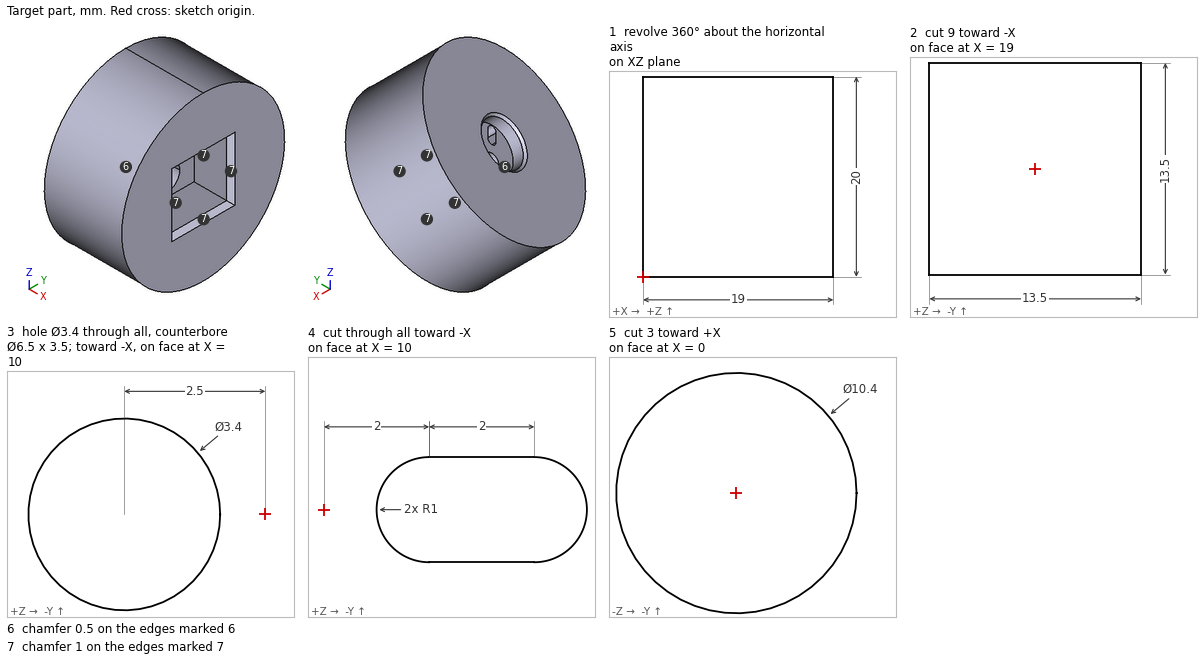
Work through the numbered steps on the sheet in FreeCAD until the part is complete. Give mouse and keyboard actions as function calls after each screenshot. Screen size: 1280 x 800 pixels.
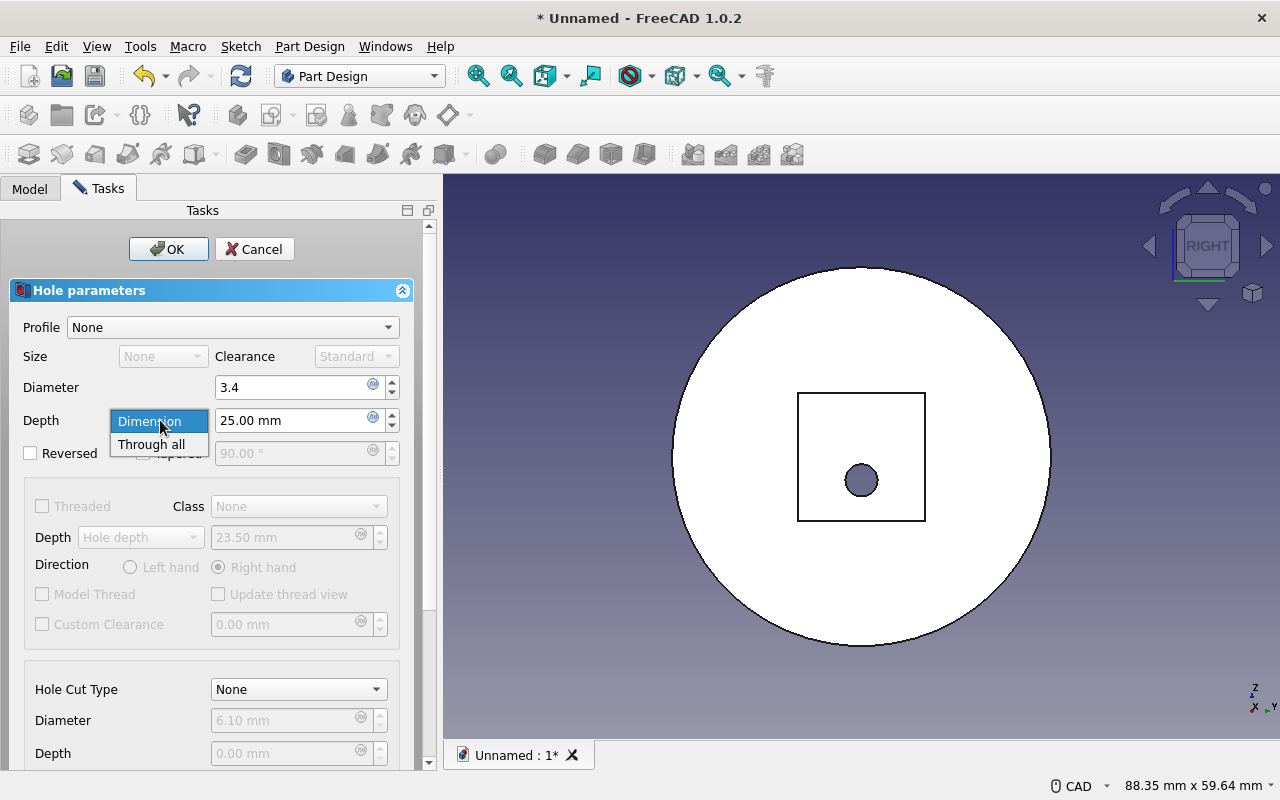
click(158, 444)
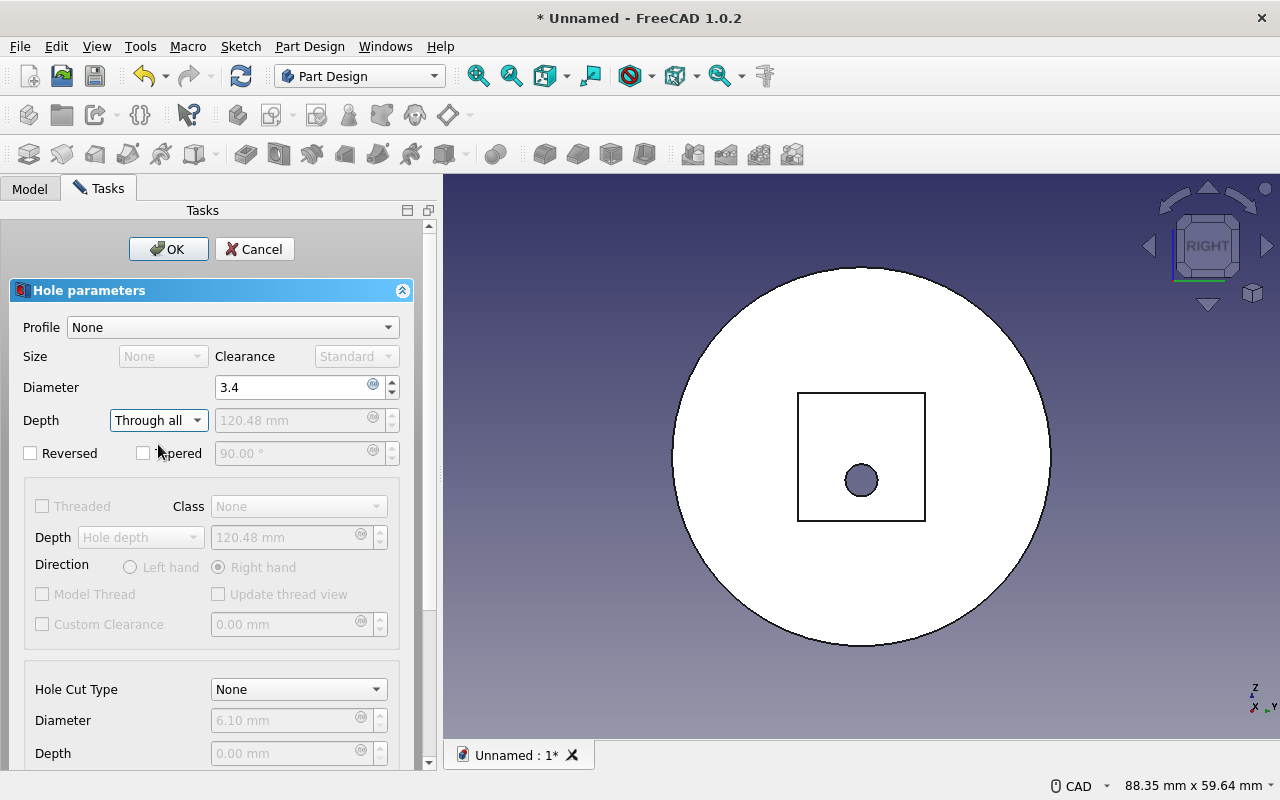
click(300, 690)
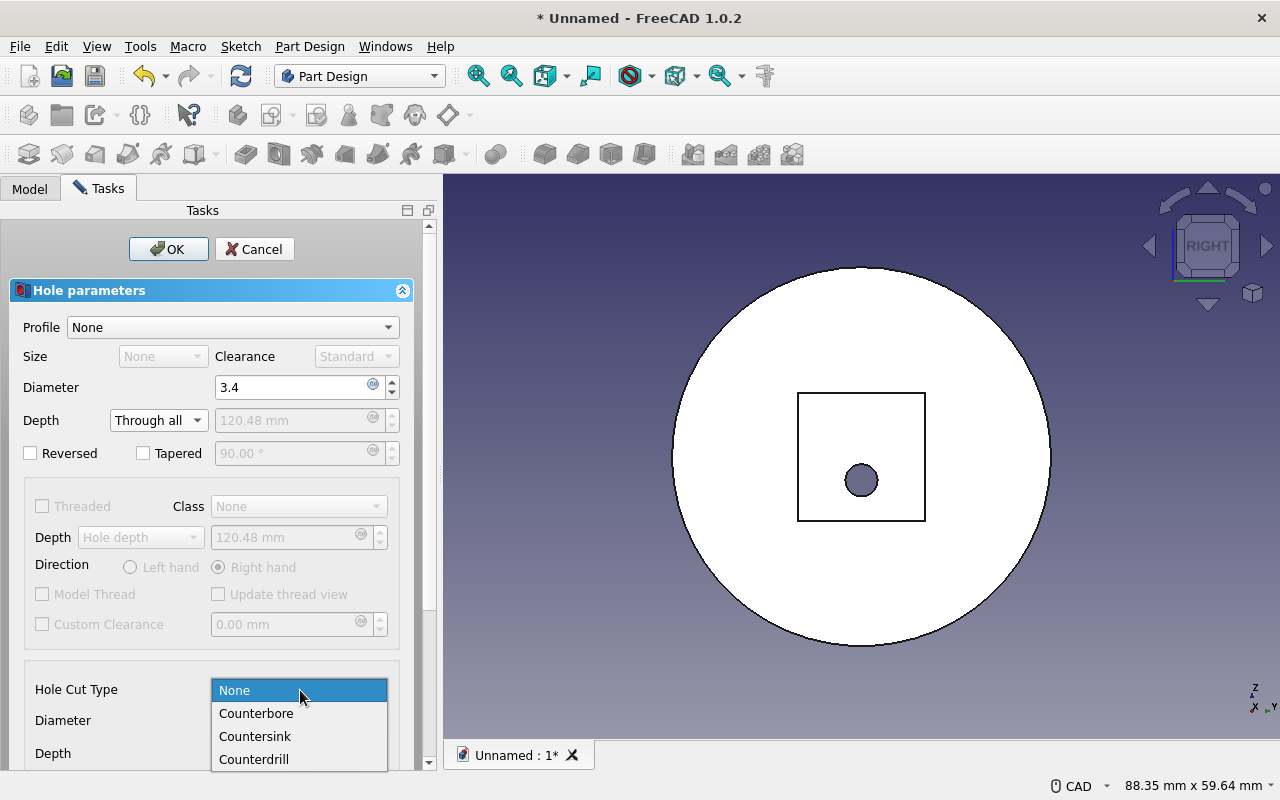
click(298, 714)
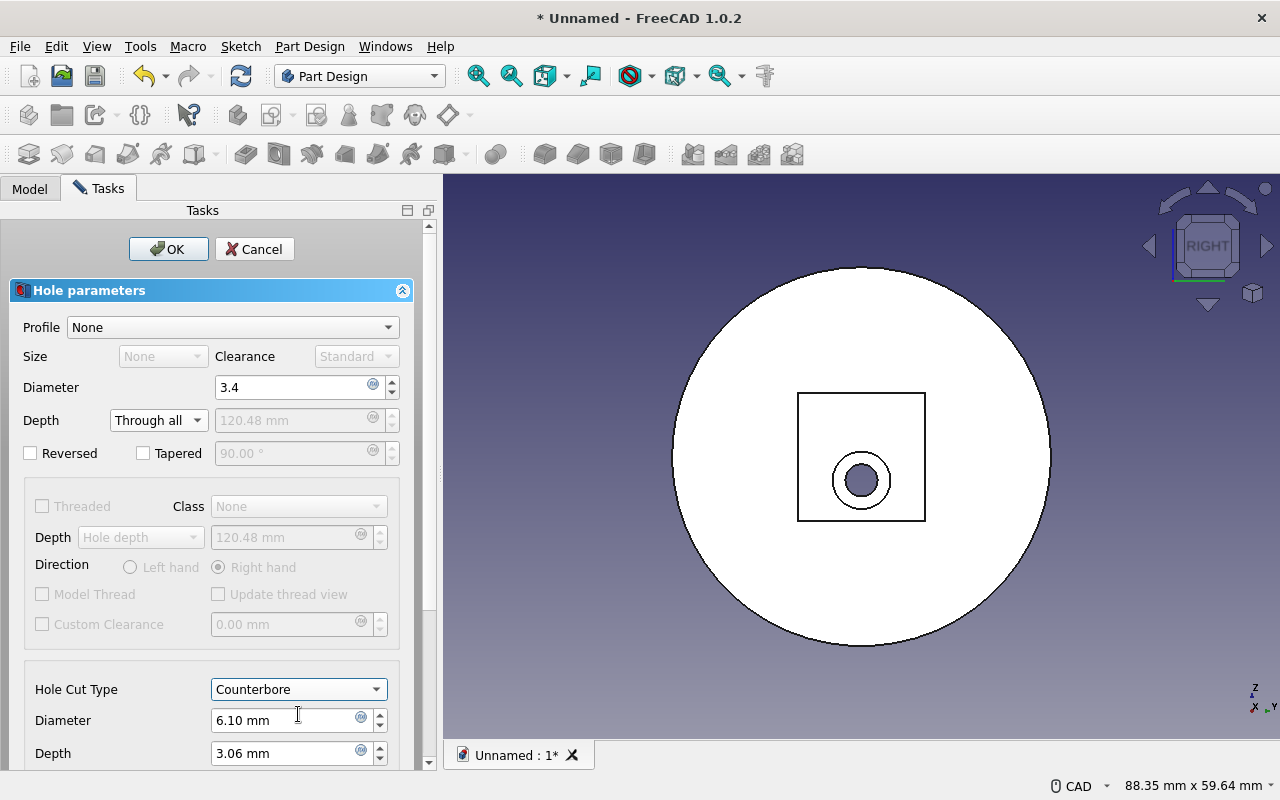
triple_click(292, 720)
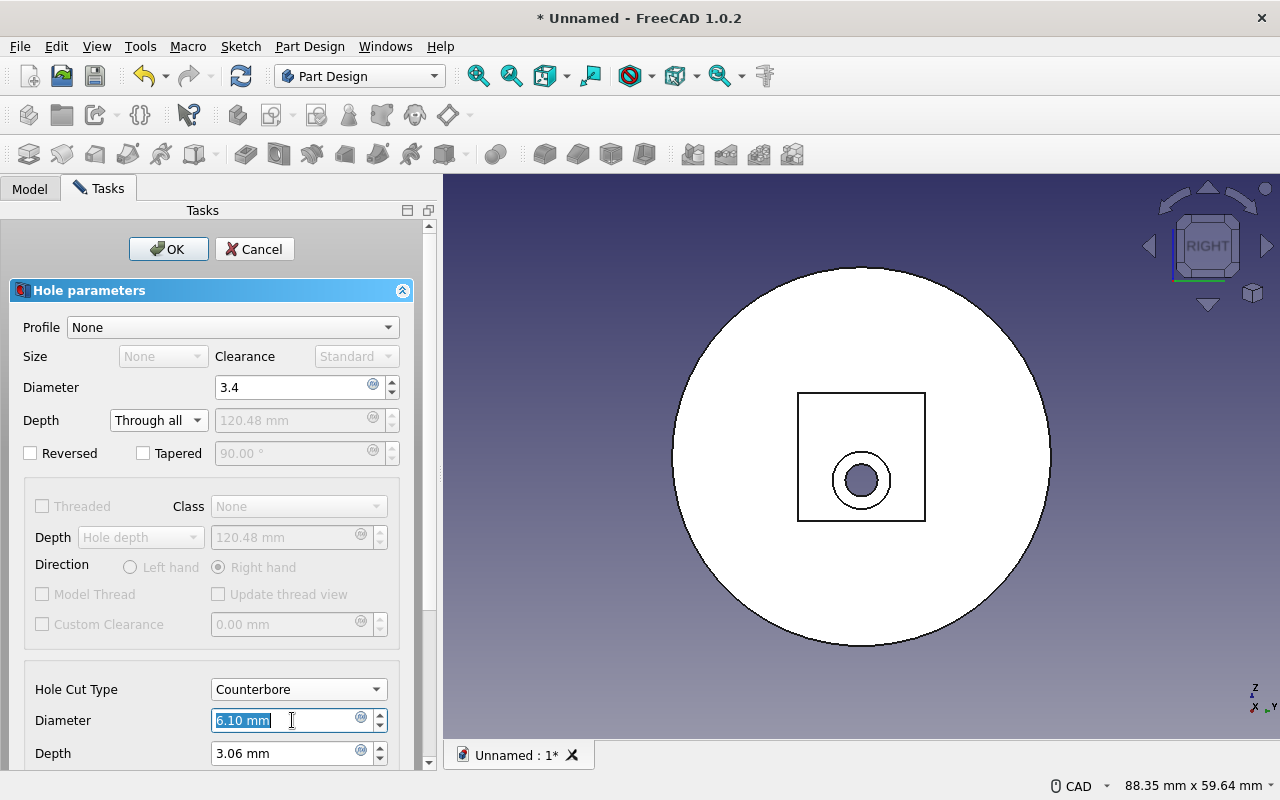
text(6.5)
key(Tab)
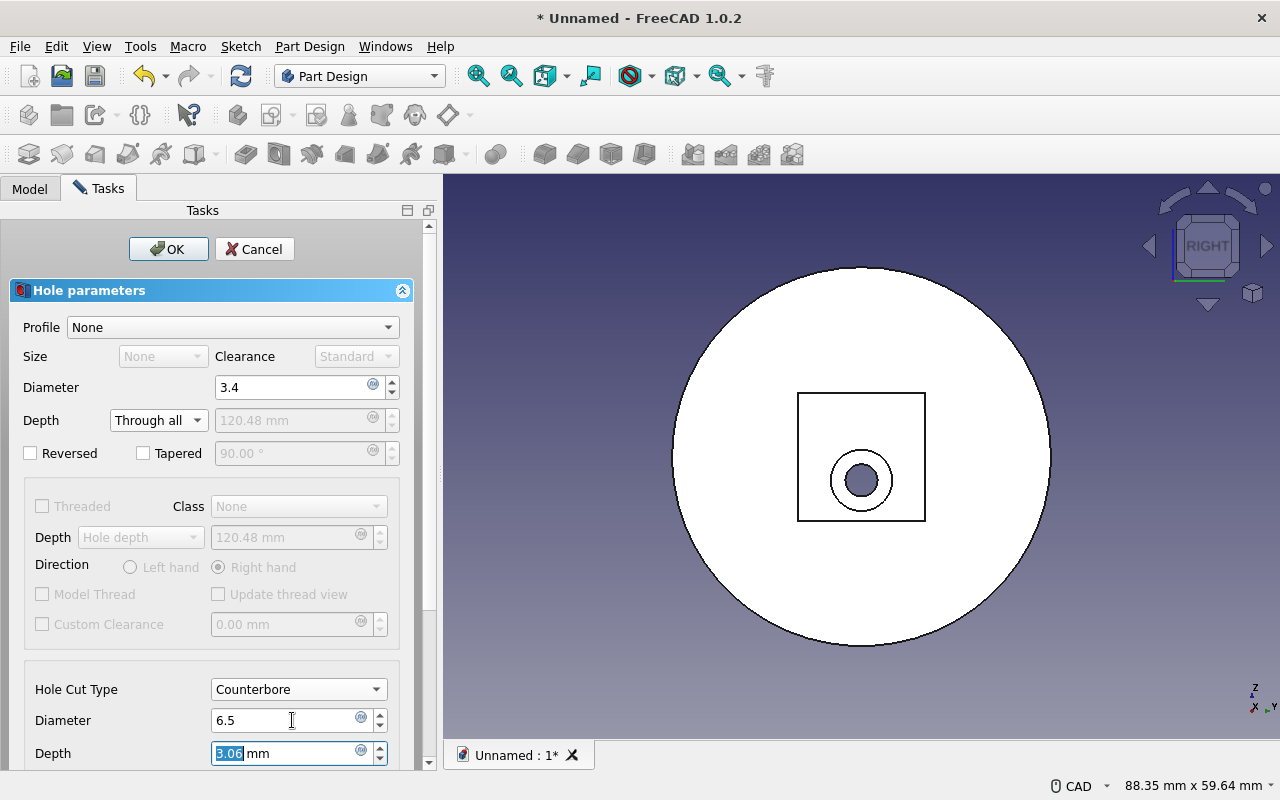
text(3.5)
key(Tab)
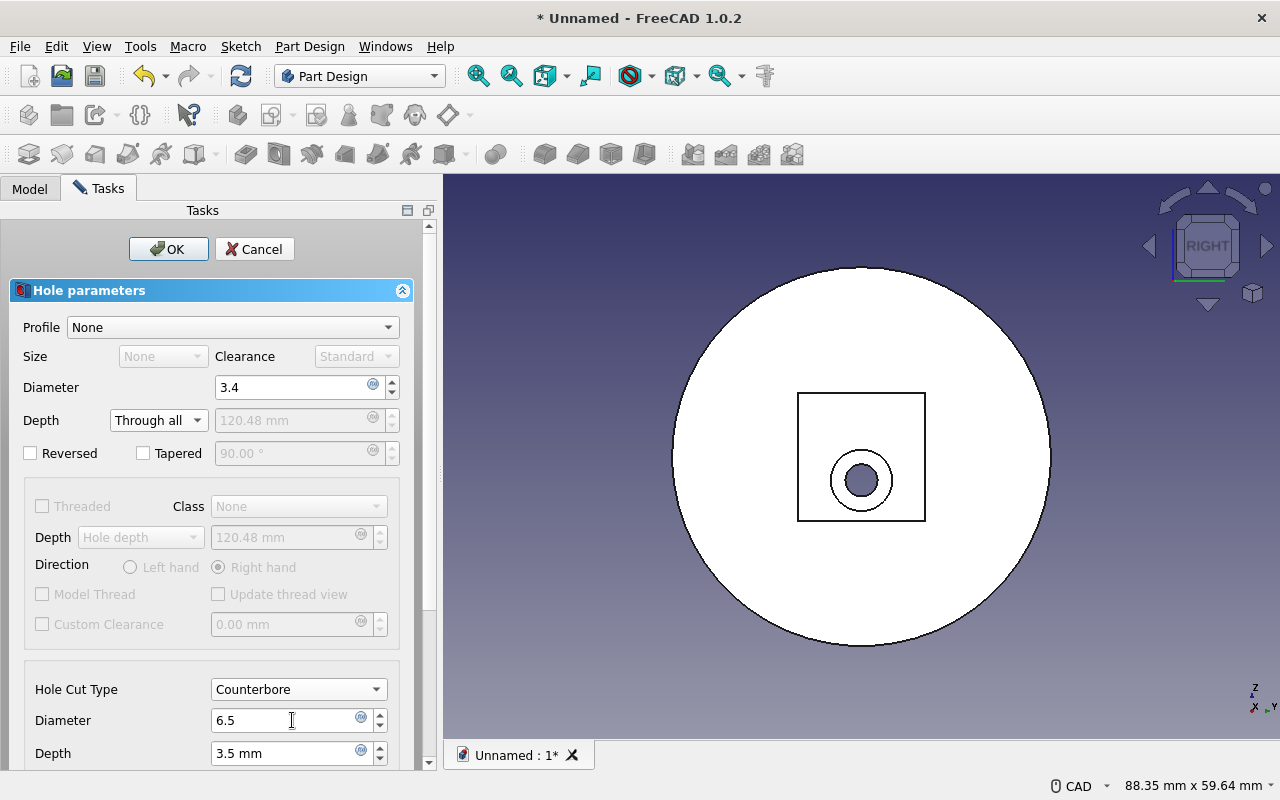
click(169, 249)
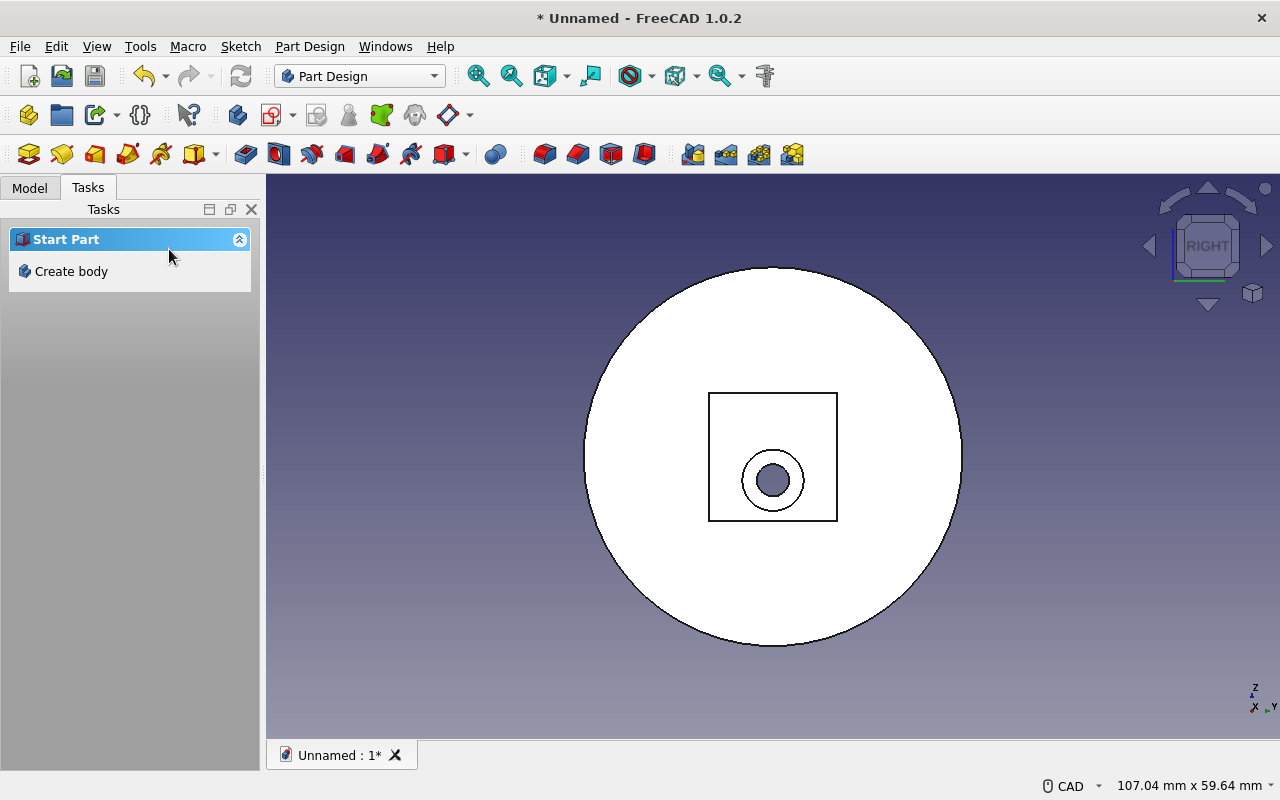
click(810, 419)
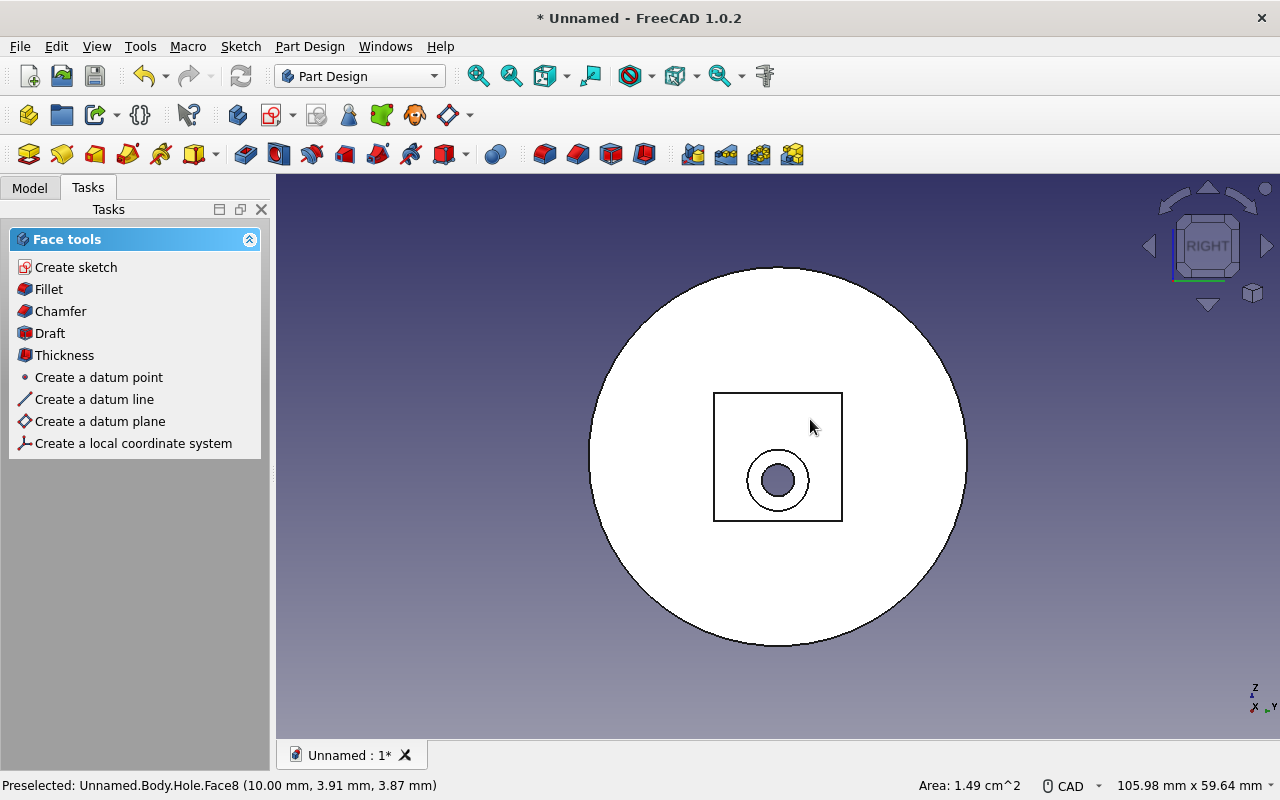
click(270, 116)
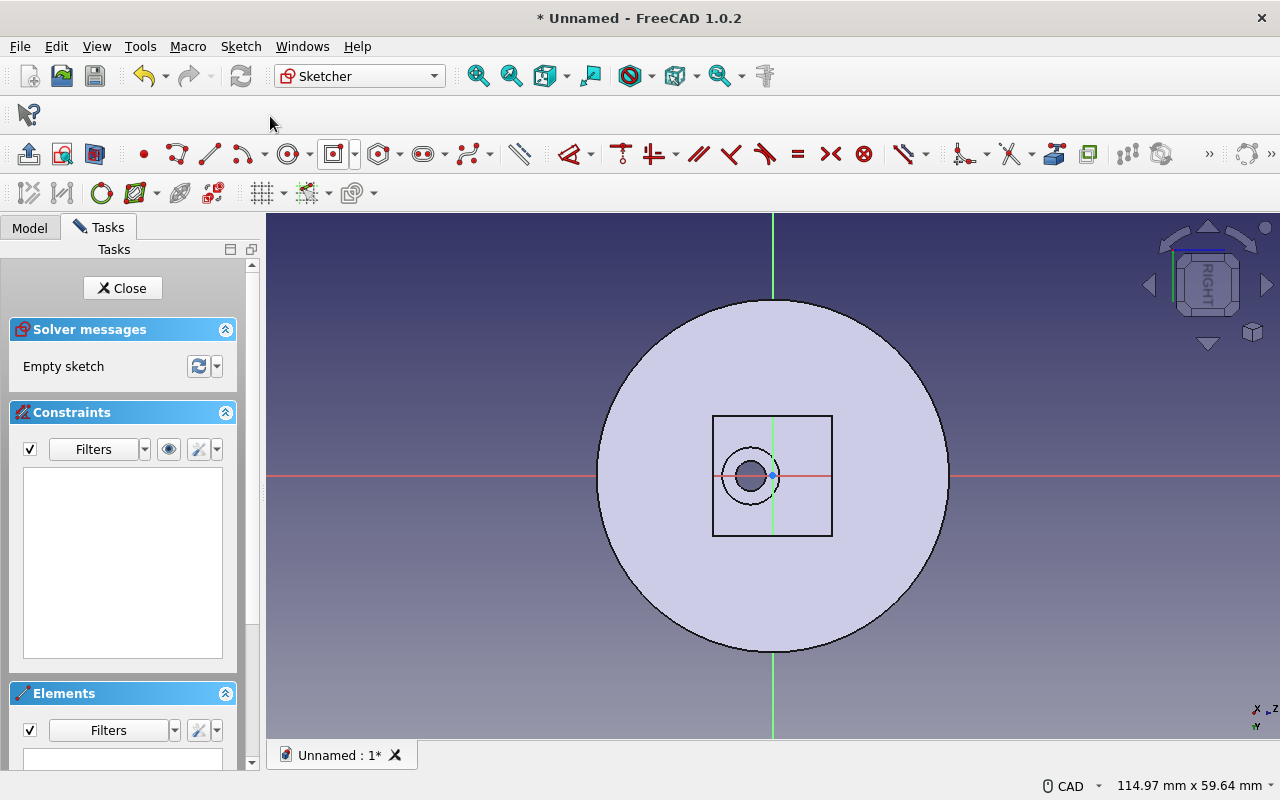
scroll(802, 476, up, 13)